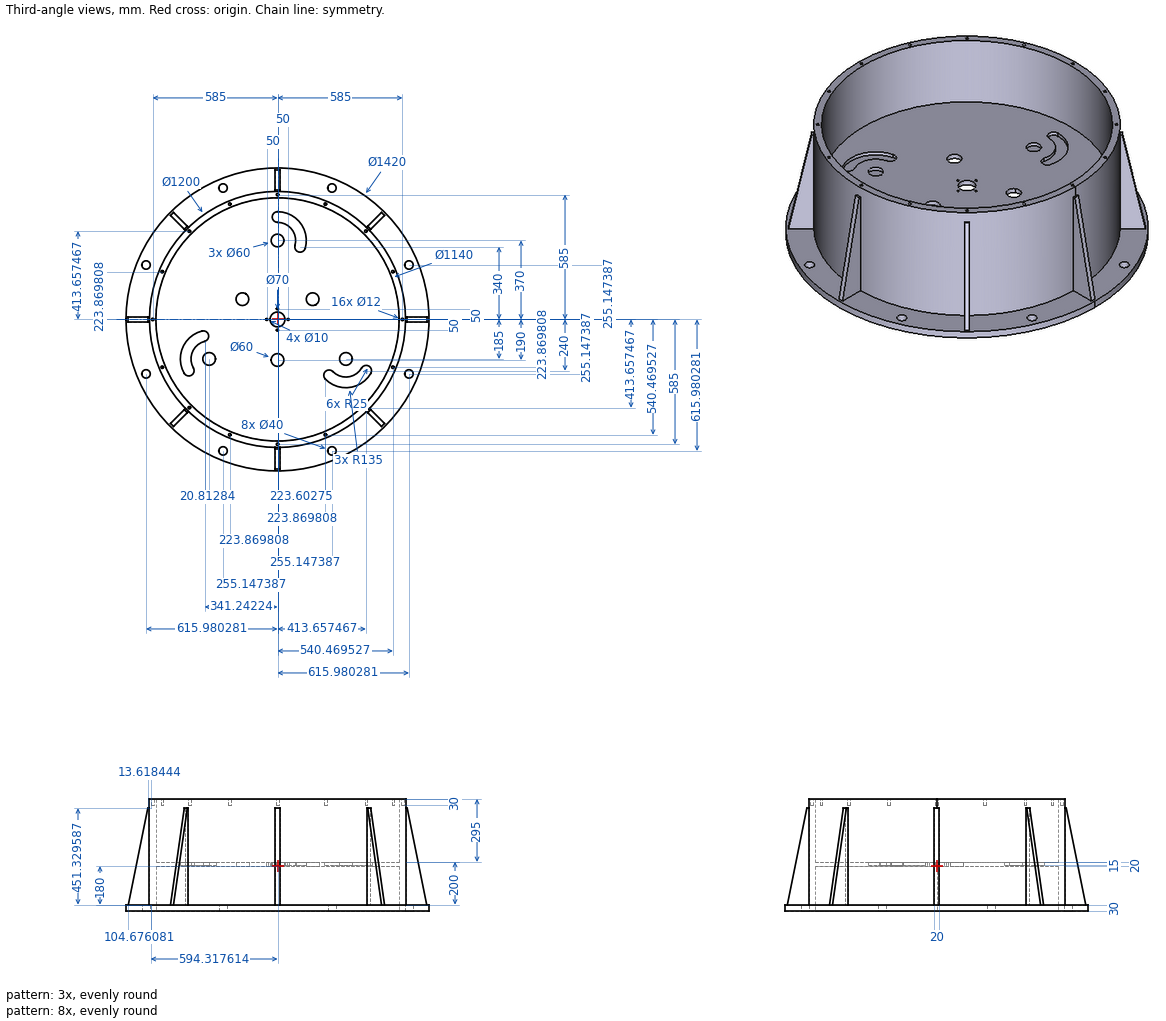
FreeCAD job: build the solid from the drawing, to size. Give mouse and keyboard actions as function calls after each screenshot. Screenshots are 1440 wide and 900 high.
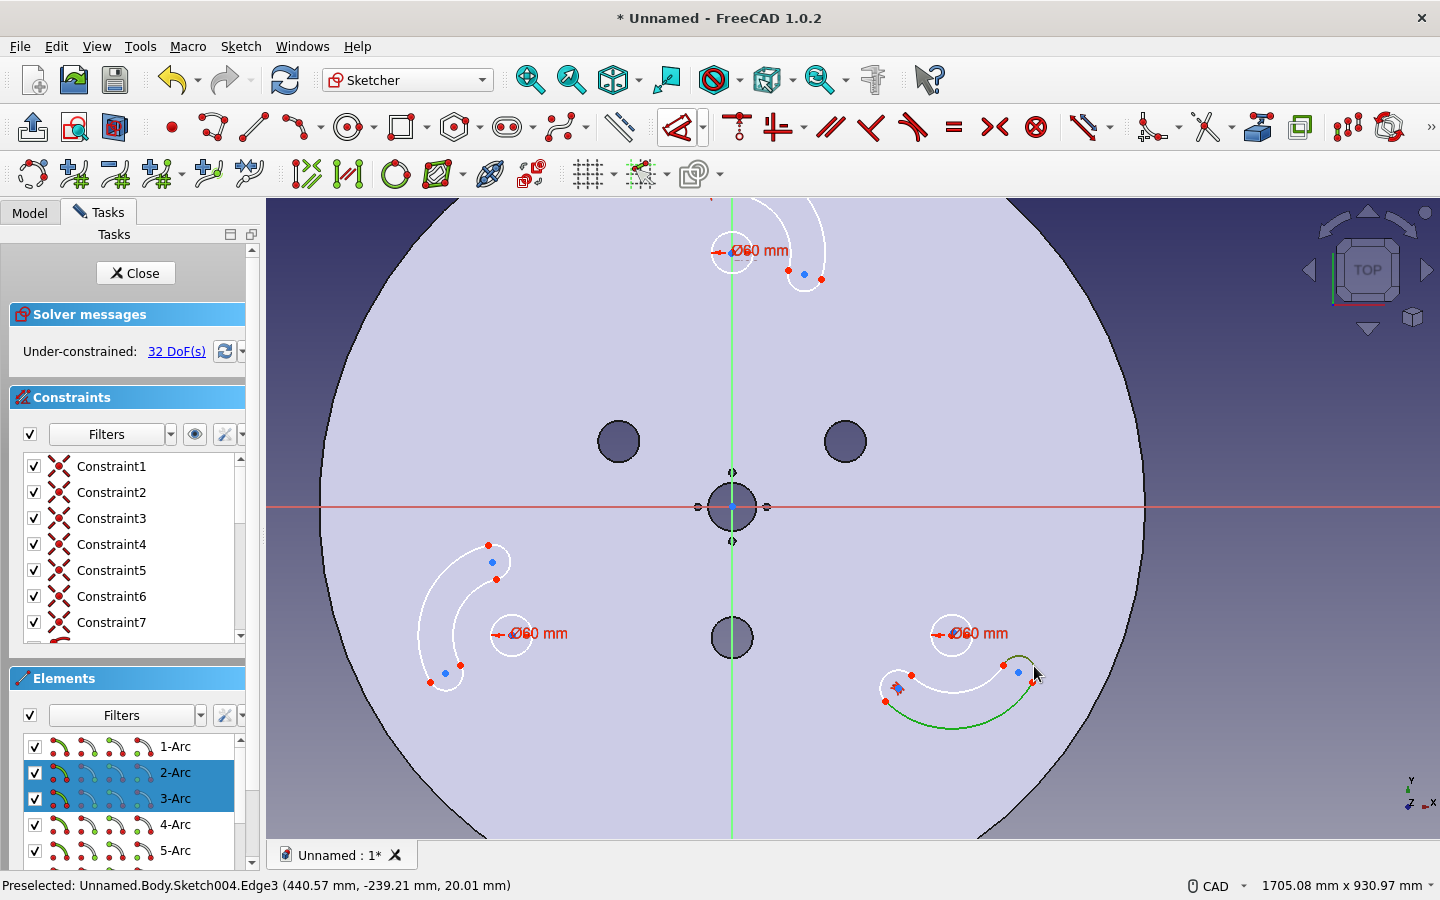
key(t)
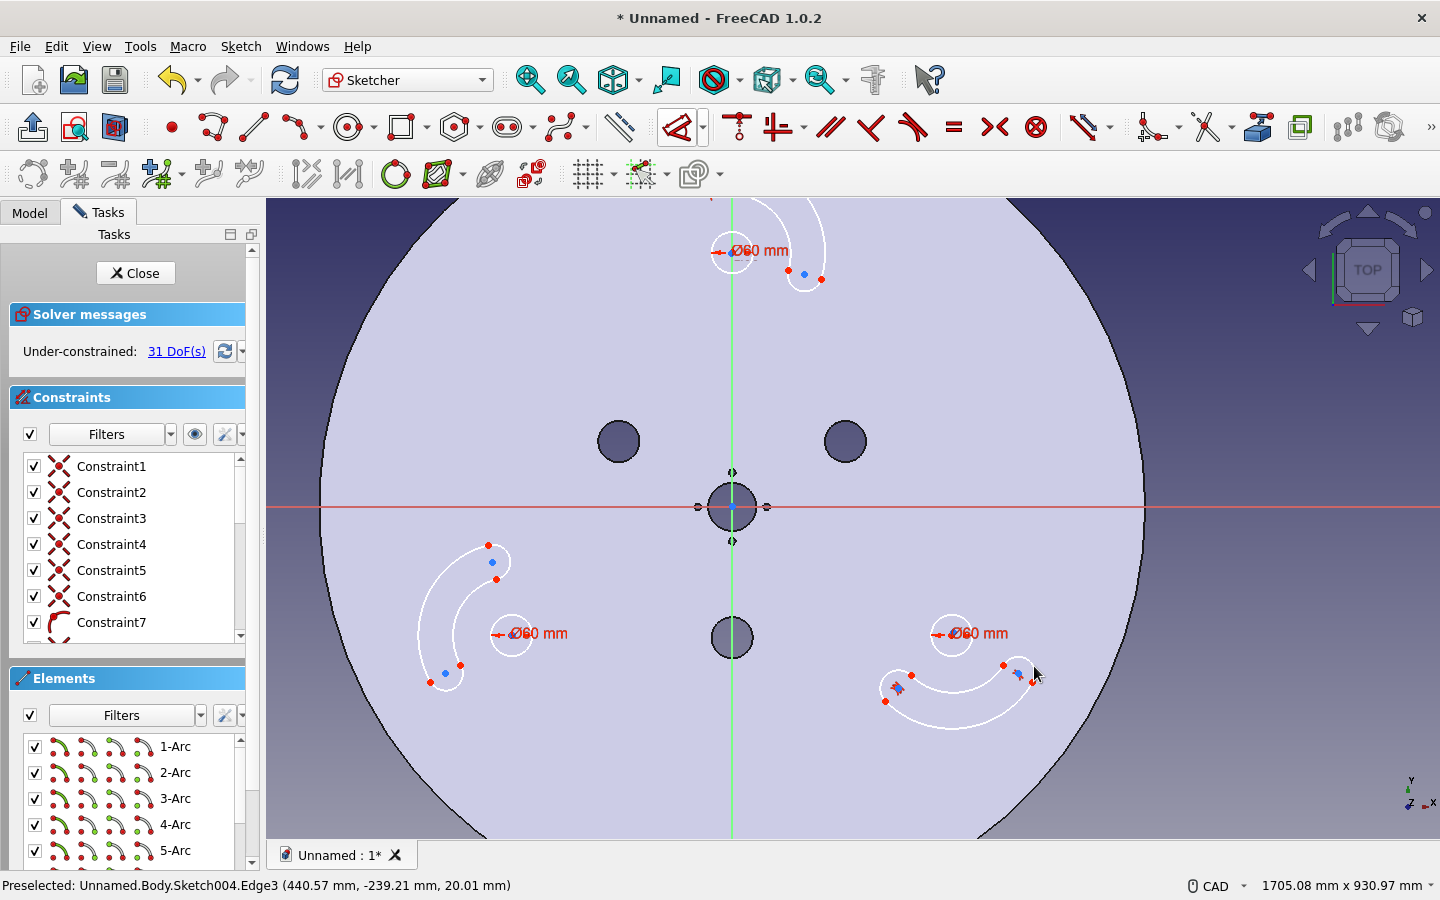
click(1034, 667)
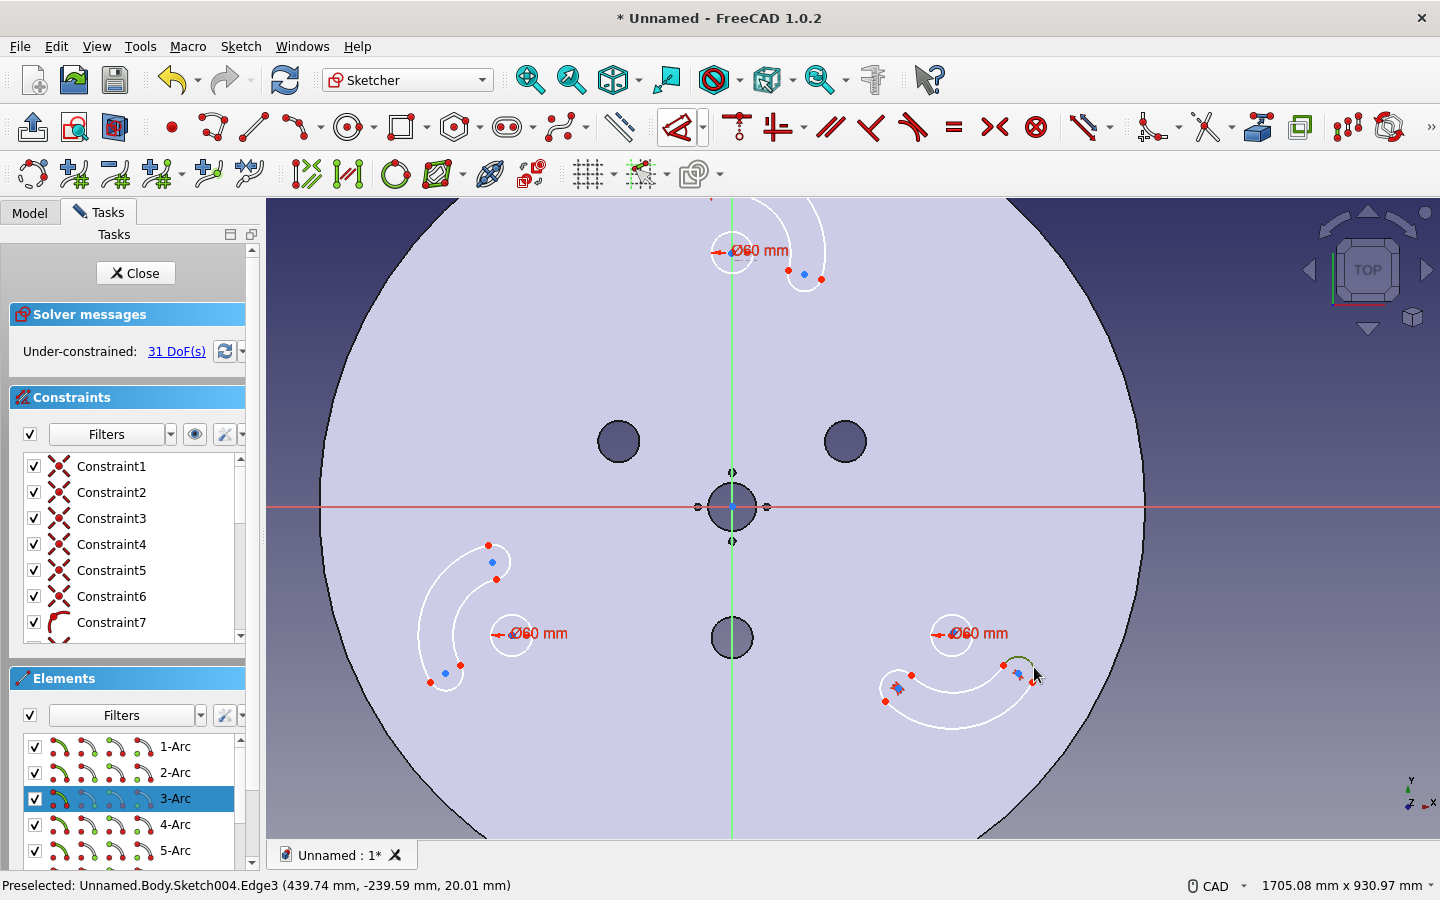
click(939, 691)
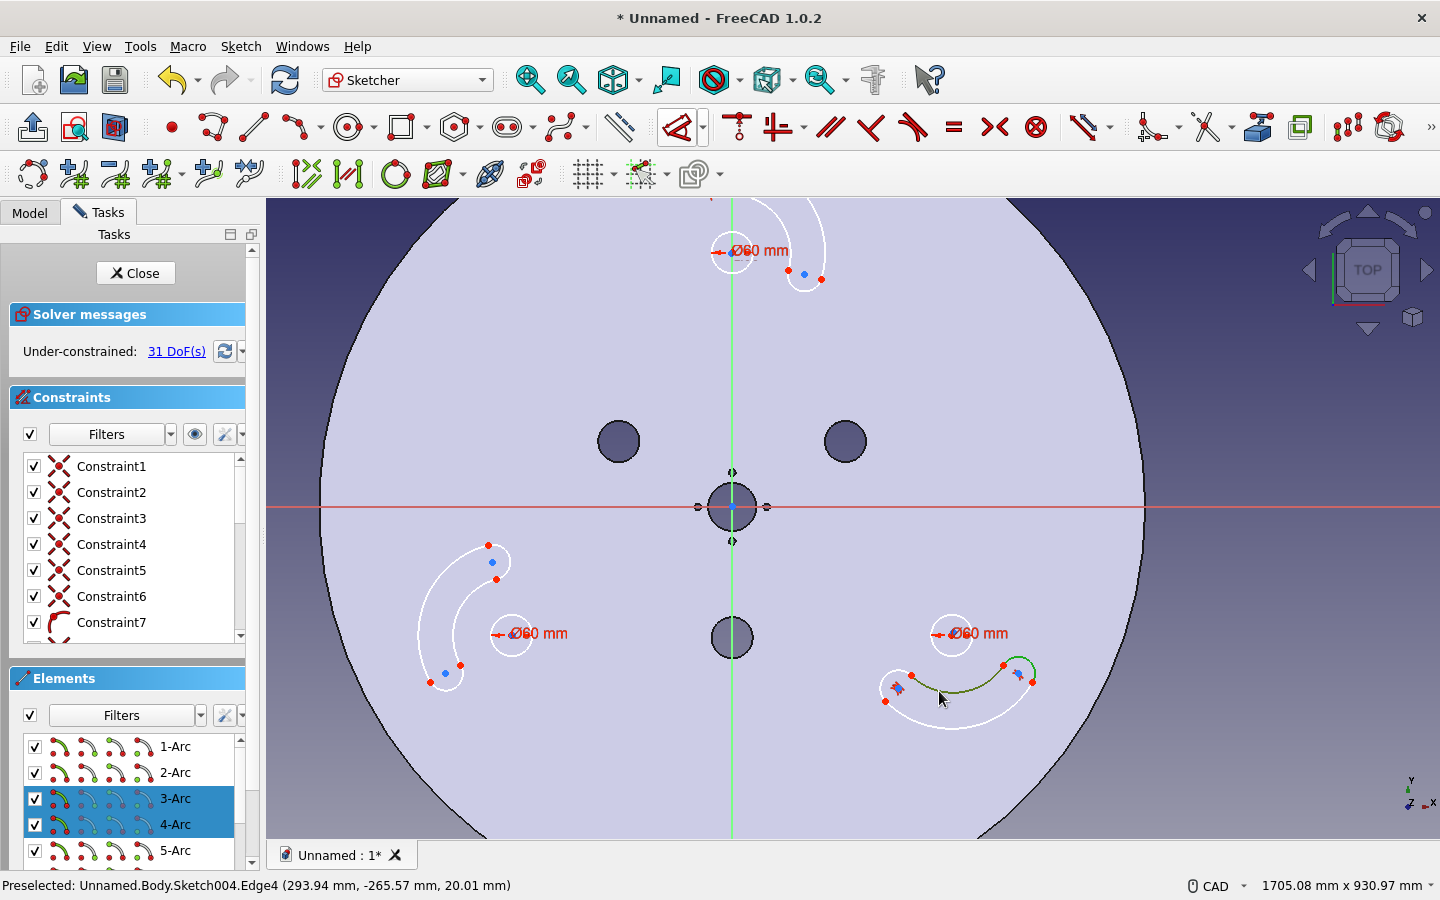
key(t)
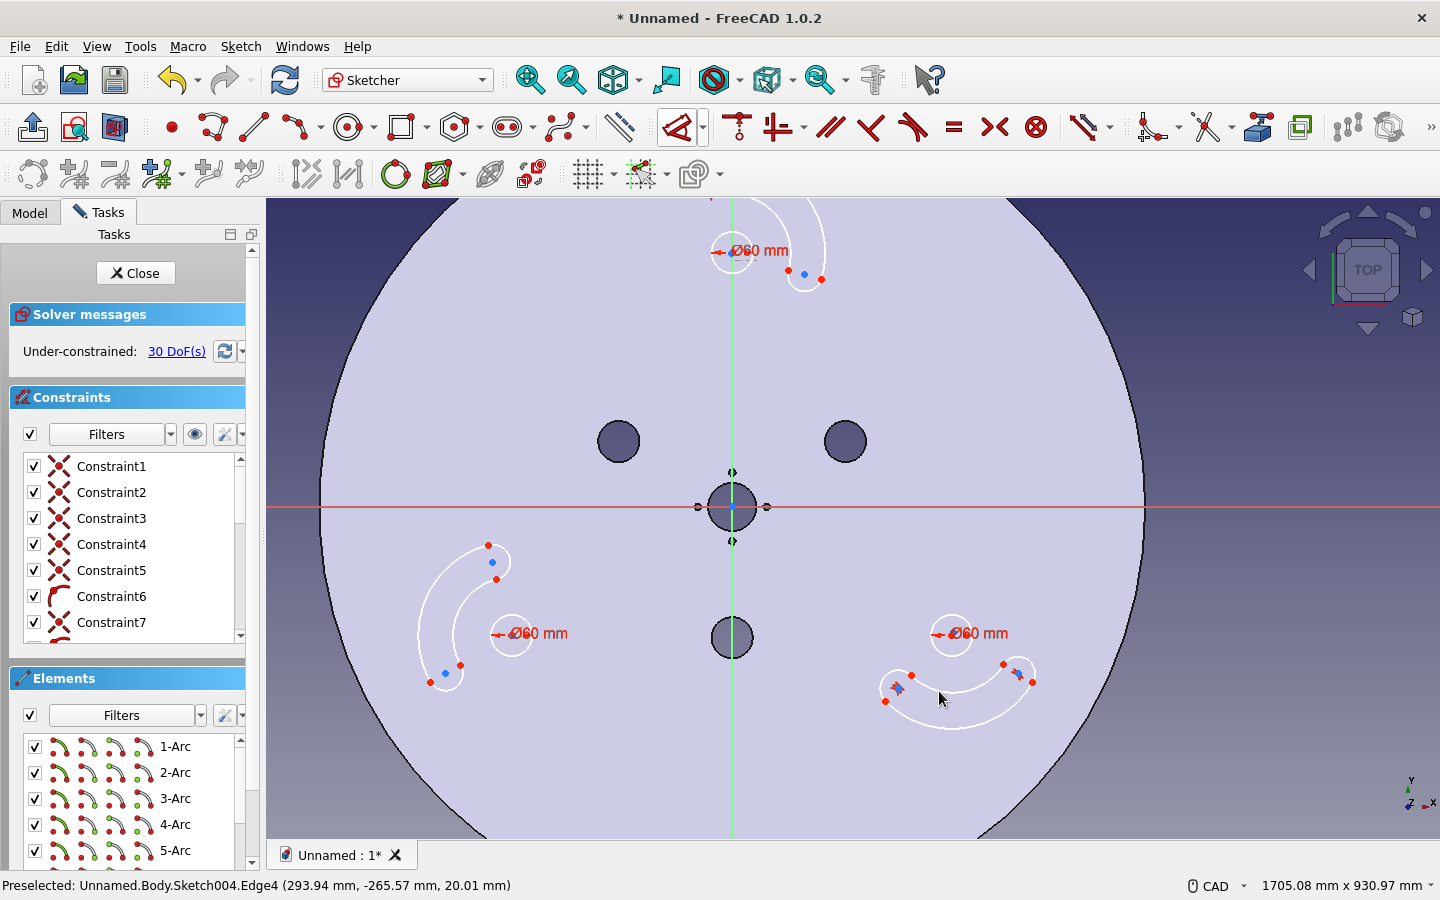
click(509, 569)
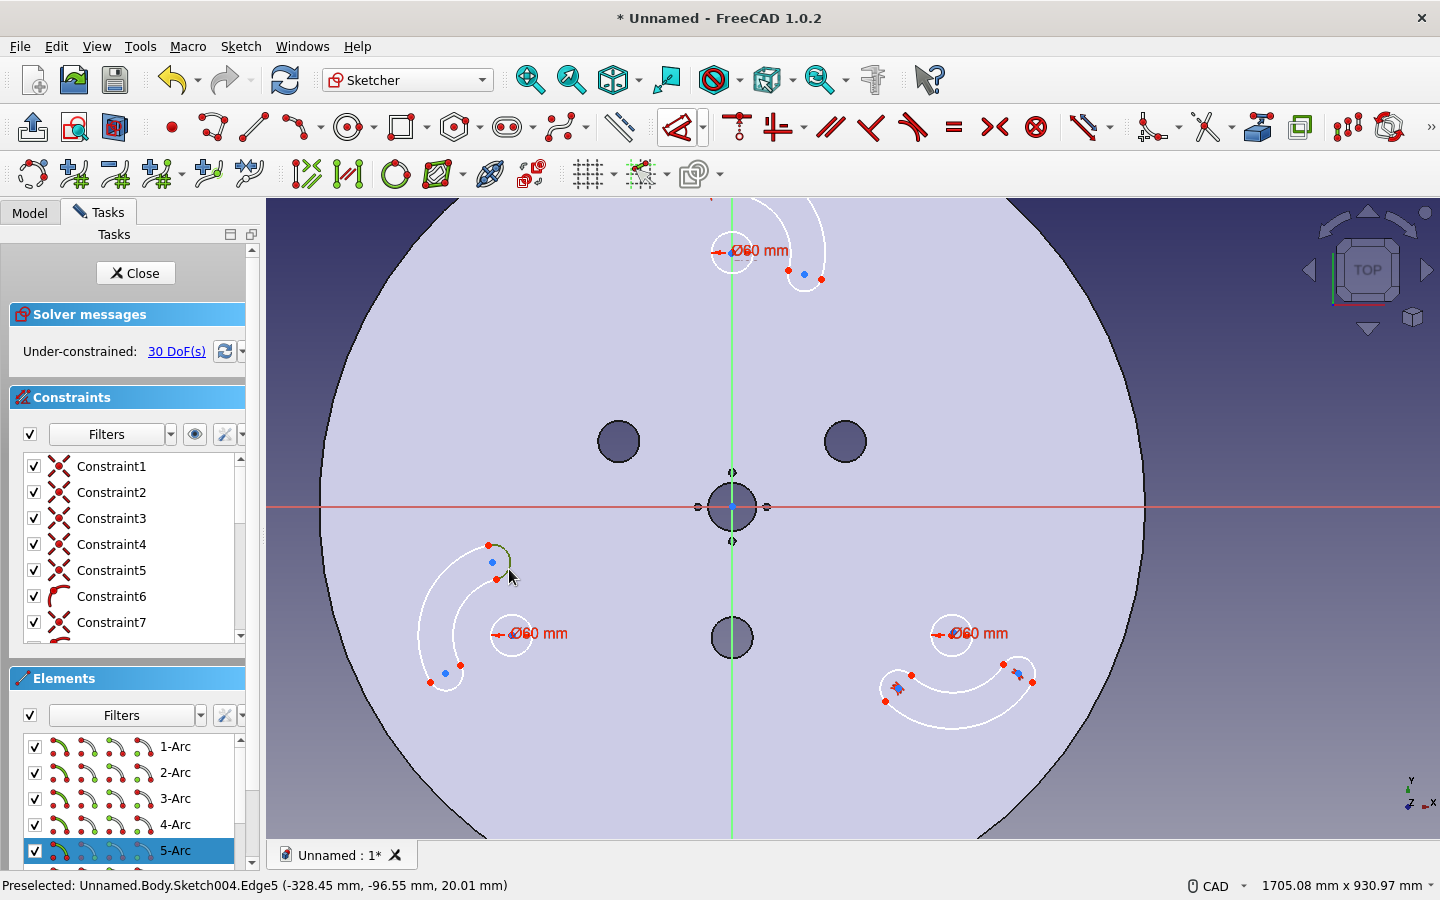
click(445, 571)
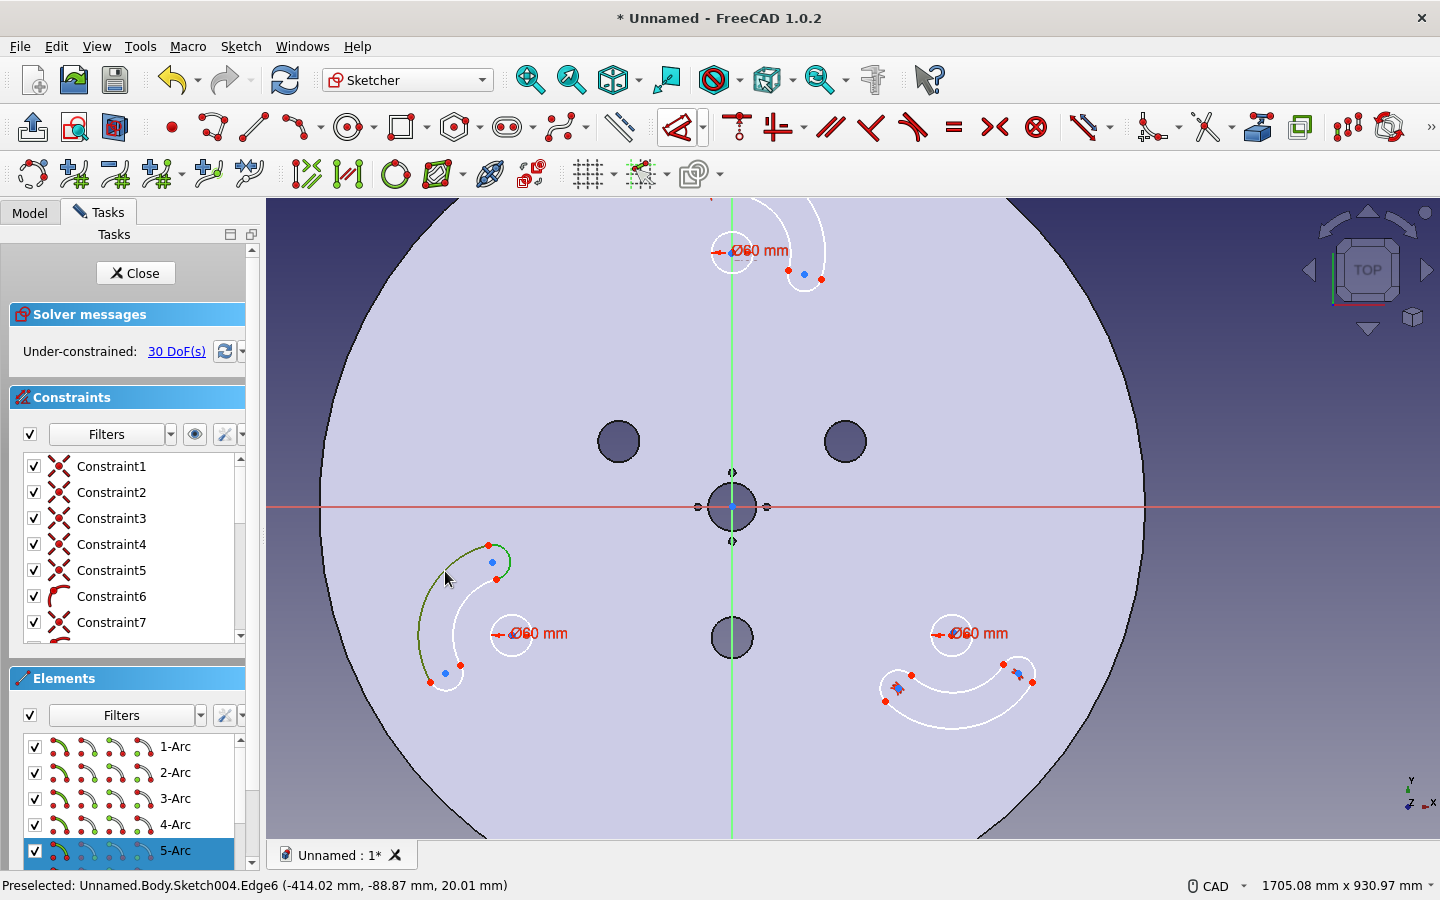
key(t)